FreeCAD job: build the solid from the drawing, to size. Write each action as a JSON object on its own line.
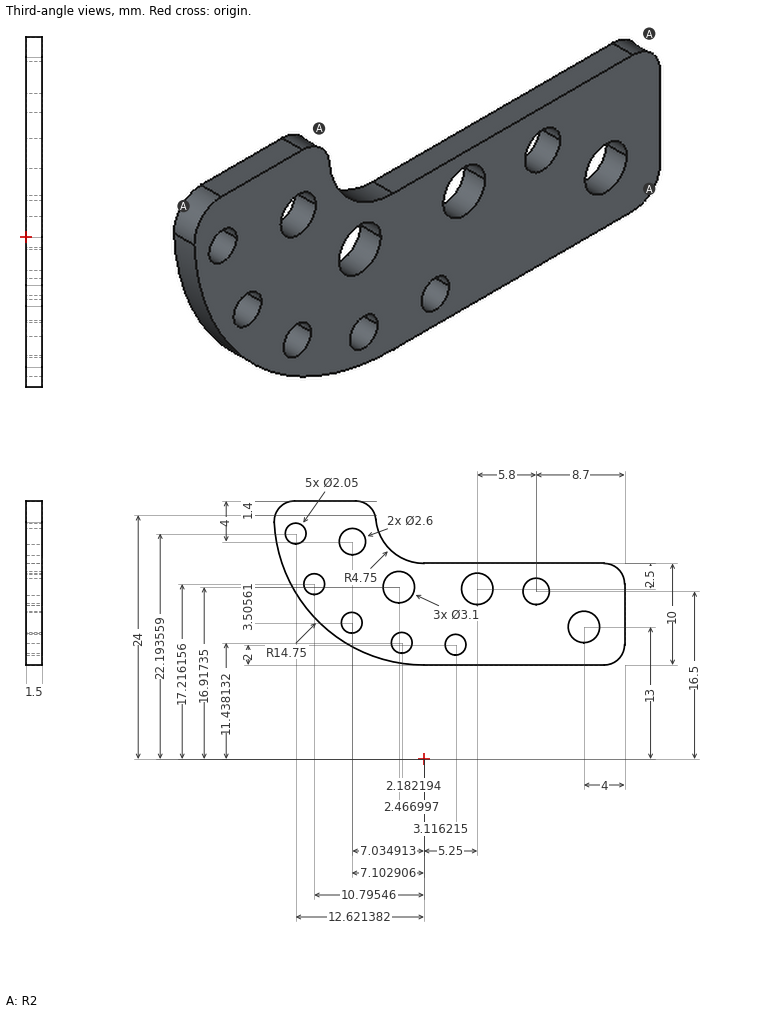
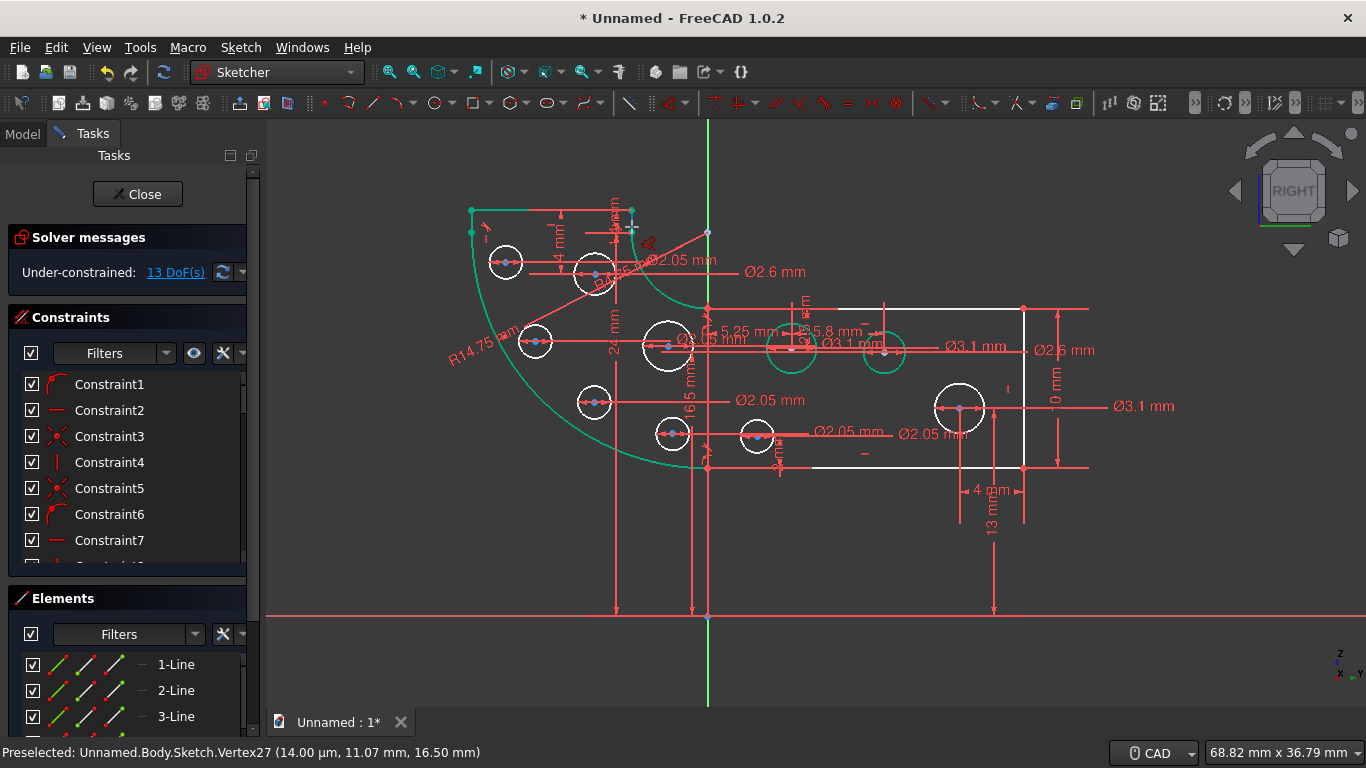
{"action": "left_click", "coordinate": [1024, 309]}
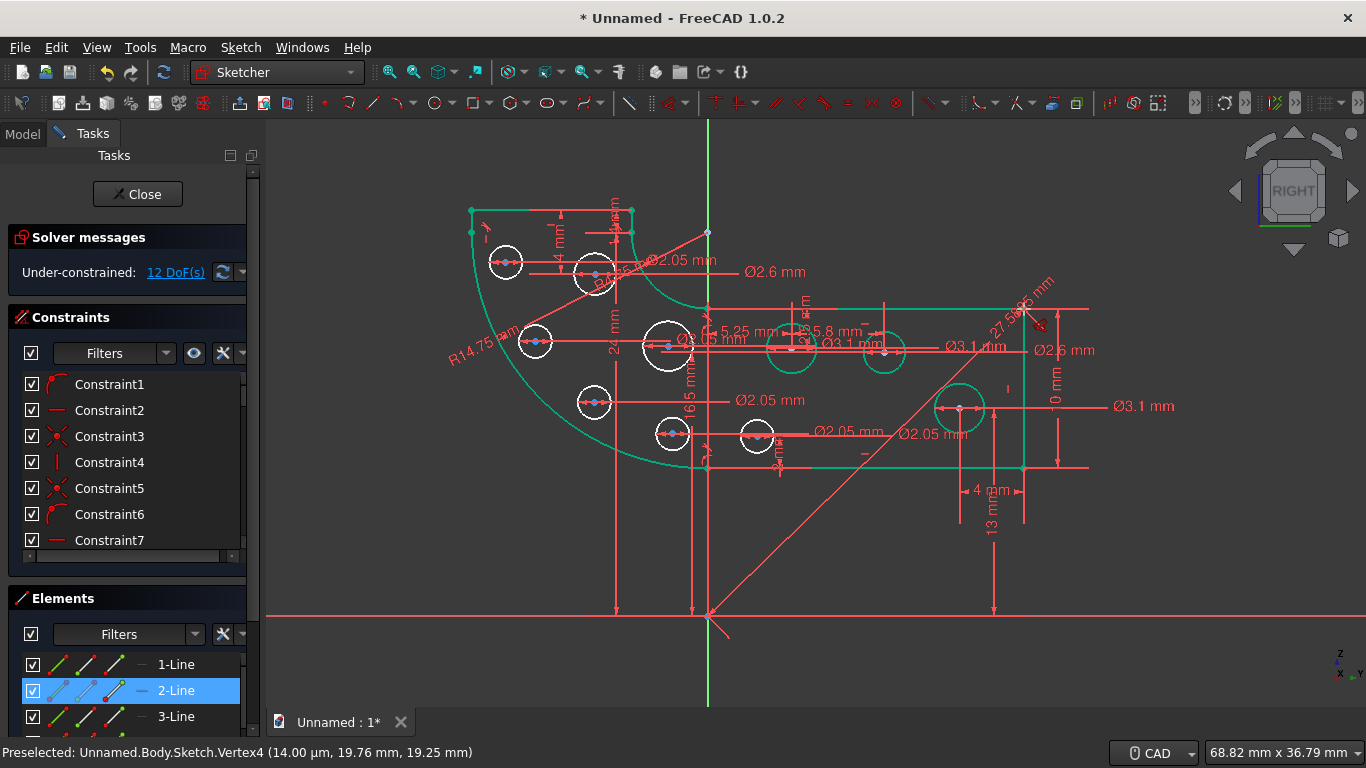
{"action": "left_click", "coordinate": [884, 352]}
{"action": "left_click", "coordinate": [954, 275]}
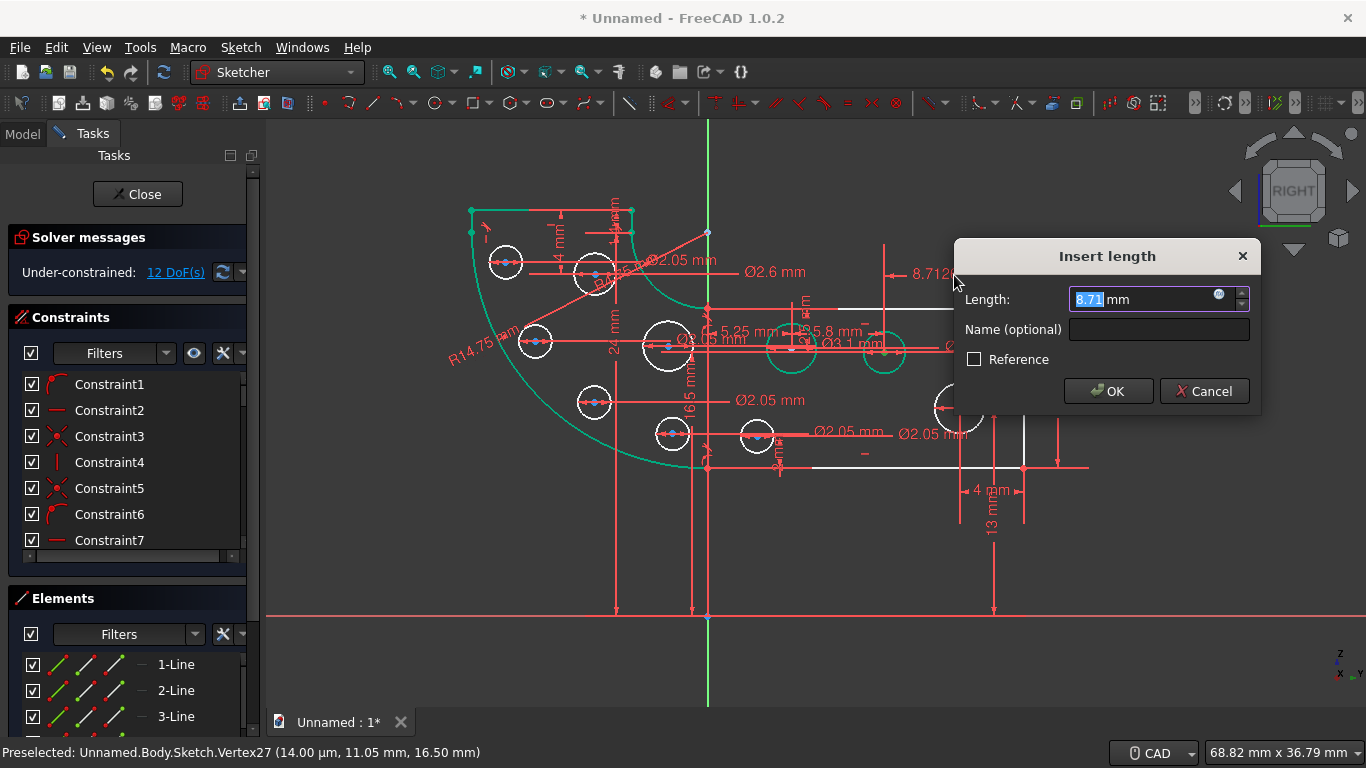
{"action": "type", "text": "8.7"}
{"action": "key", "text": "Return"}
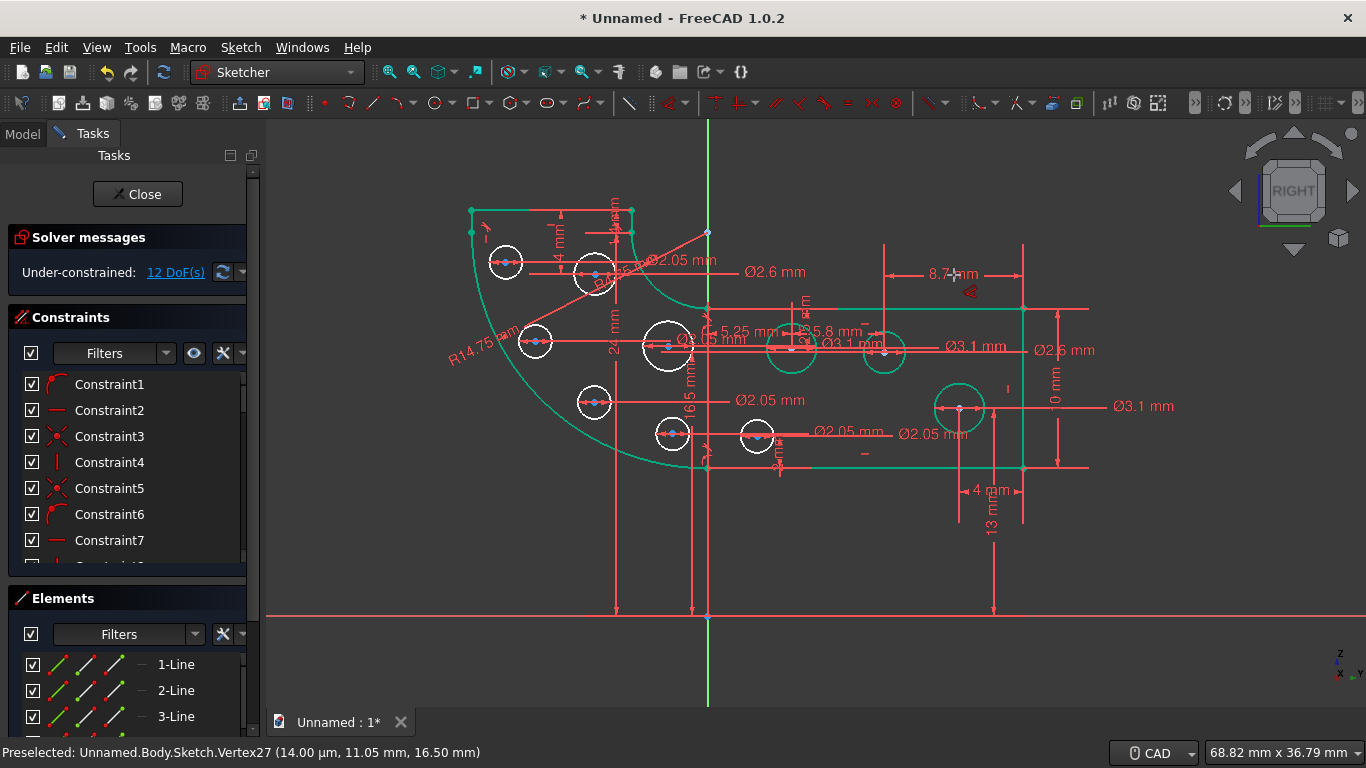
{"action": "left_click", "coordinate": [595, 274]}
{"action": "left_click", "coordinate": [651, 650]}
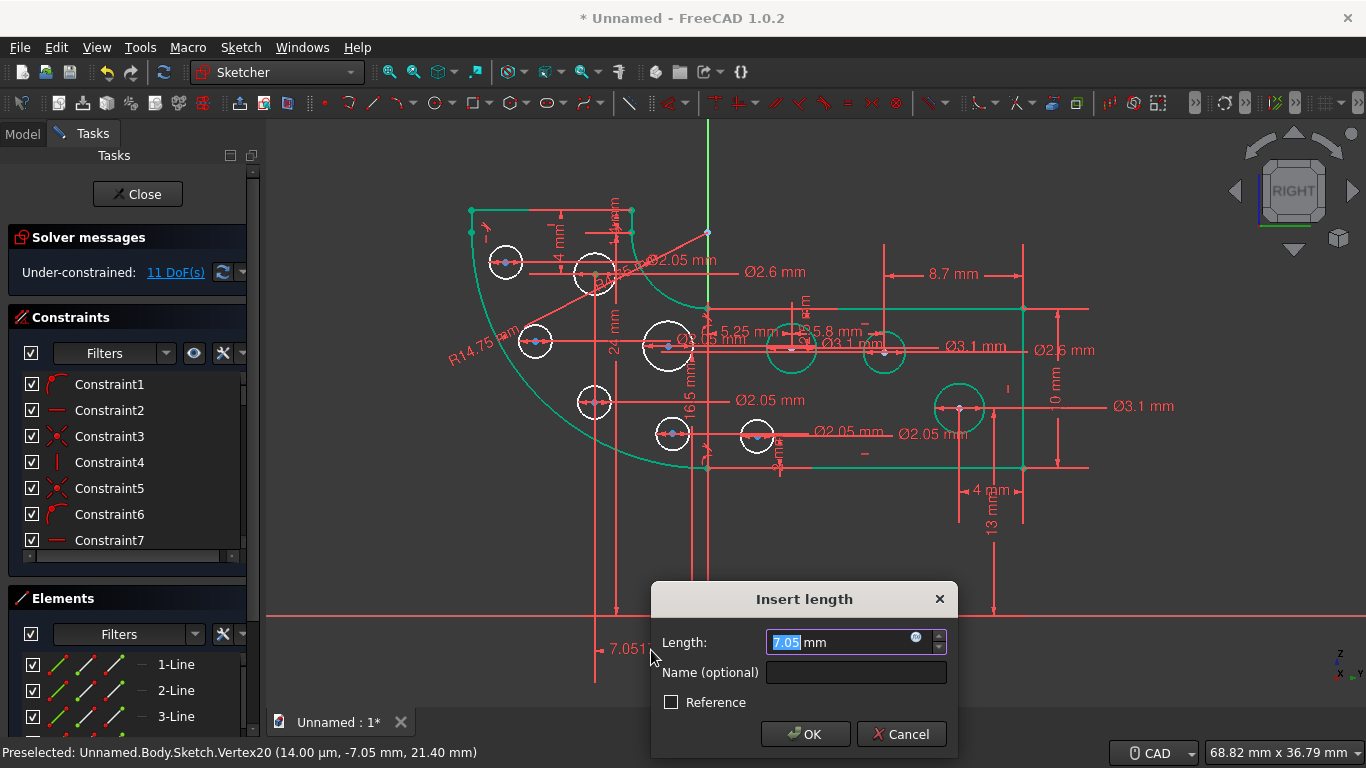
{"action": "type", "text": "7.034913"}
{"action": "key", "text": "Return"}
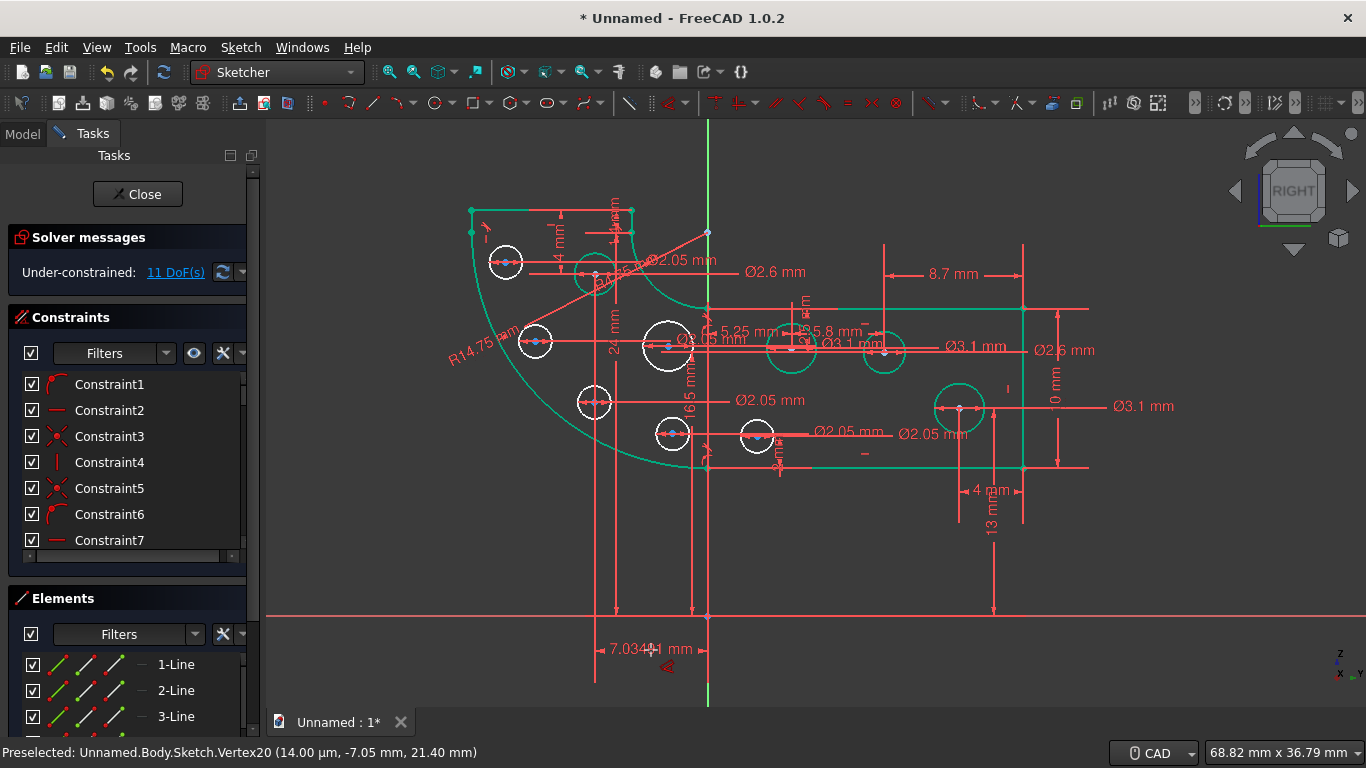
{"action": "left_click", "coordinate": [535, 341]}
{"action": "left_click", "coordinate": [561, 650]}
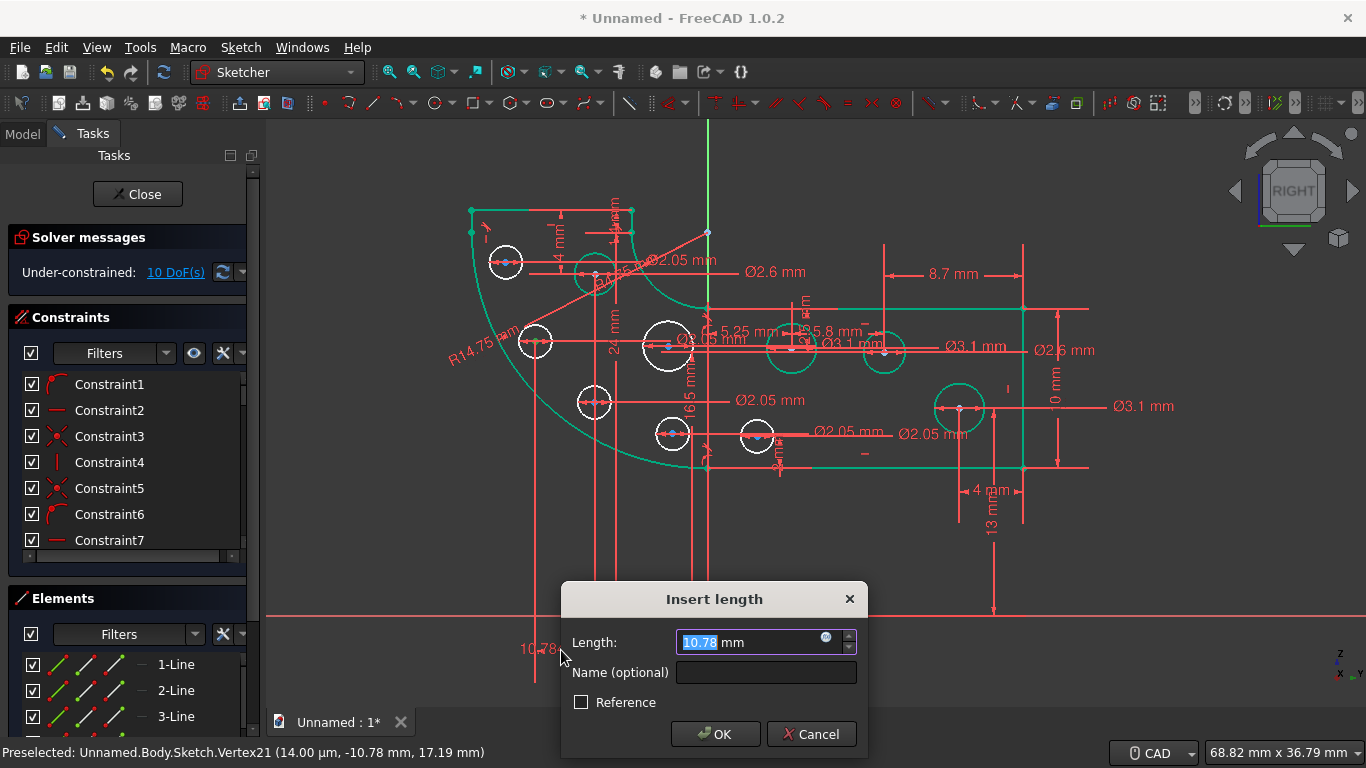
{"action": "type", "text": "10.79546"}
{"action": "key", "text": "Return"}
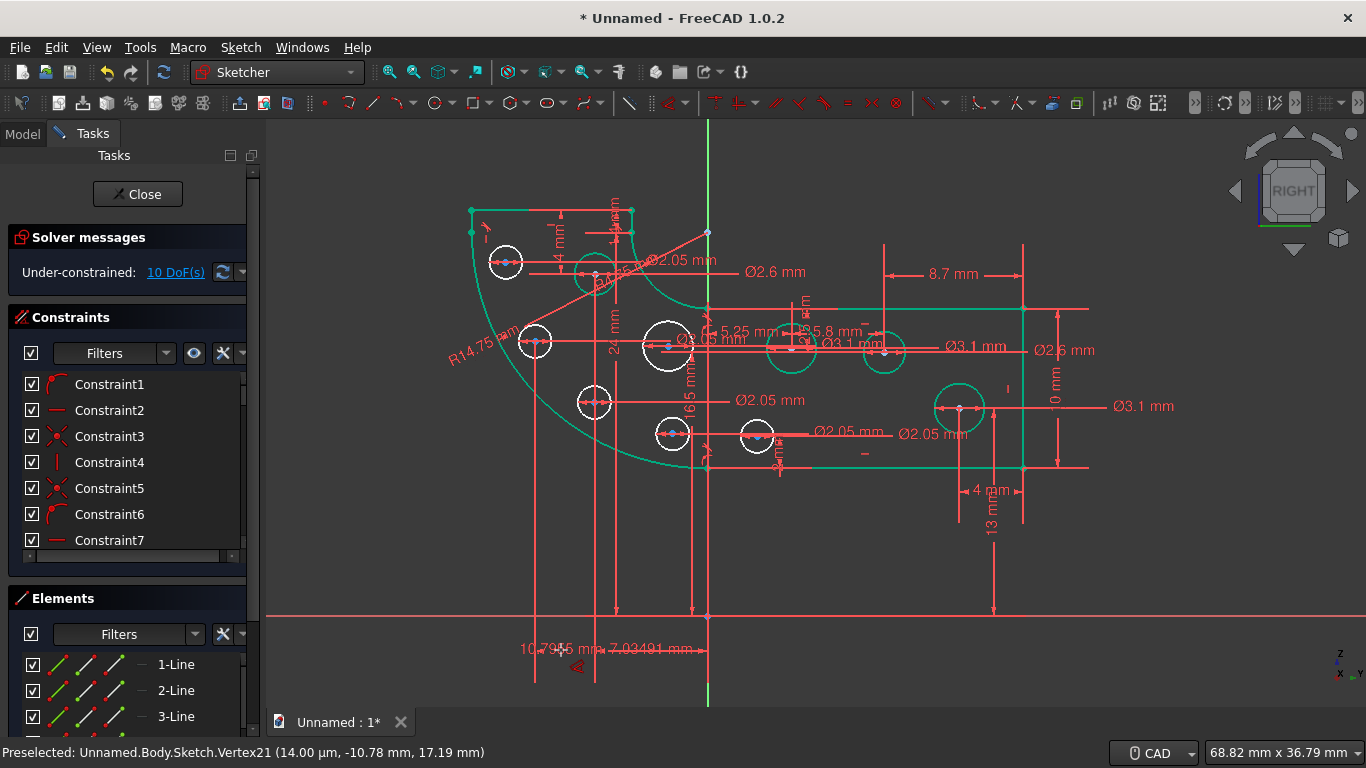
{"action": "left_click", "coordinate": [668, 346]}
{"action": "left_click", "coordinate": [688, 674]}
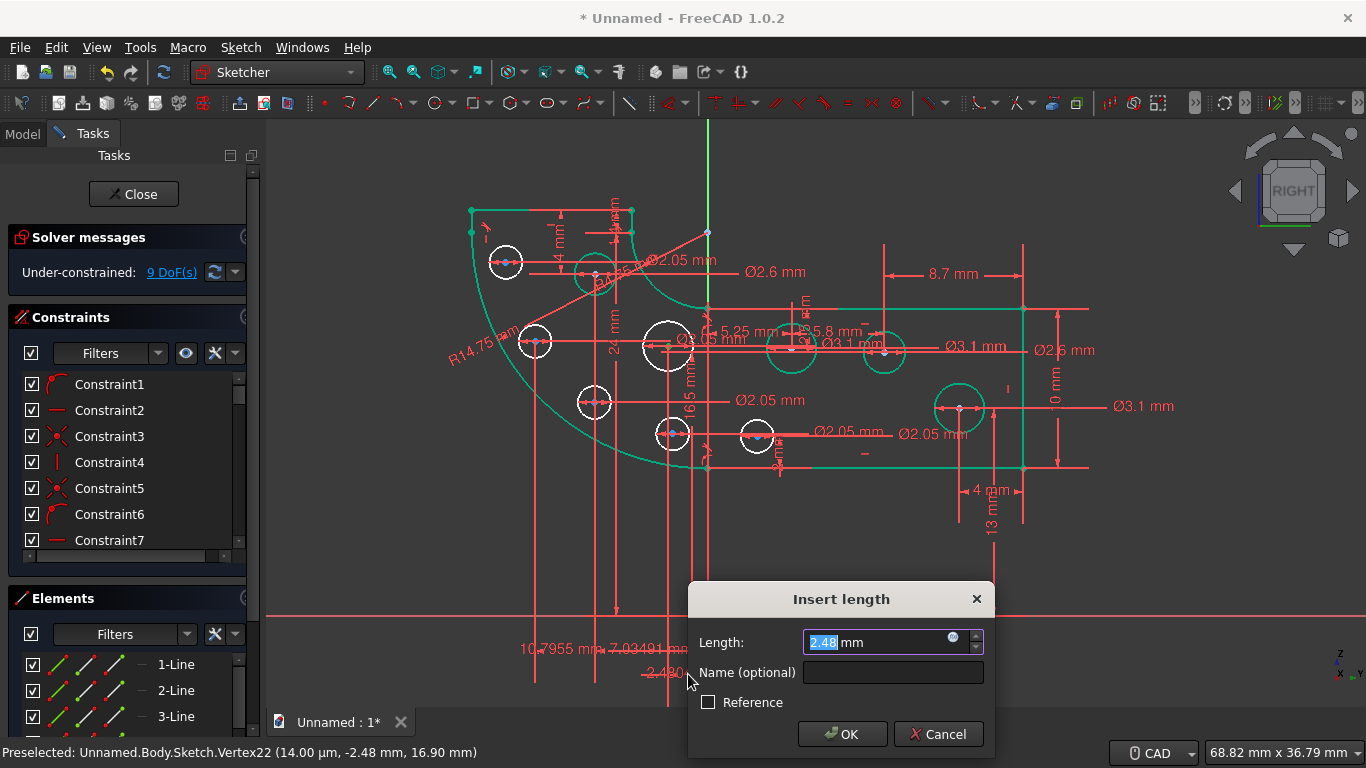
{"action": "type", "text": "2.466997"}
{"action": "key", "text": "Return"}